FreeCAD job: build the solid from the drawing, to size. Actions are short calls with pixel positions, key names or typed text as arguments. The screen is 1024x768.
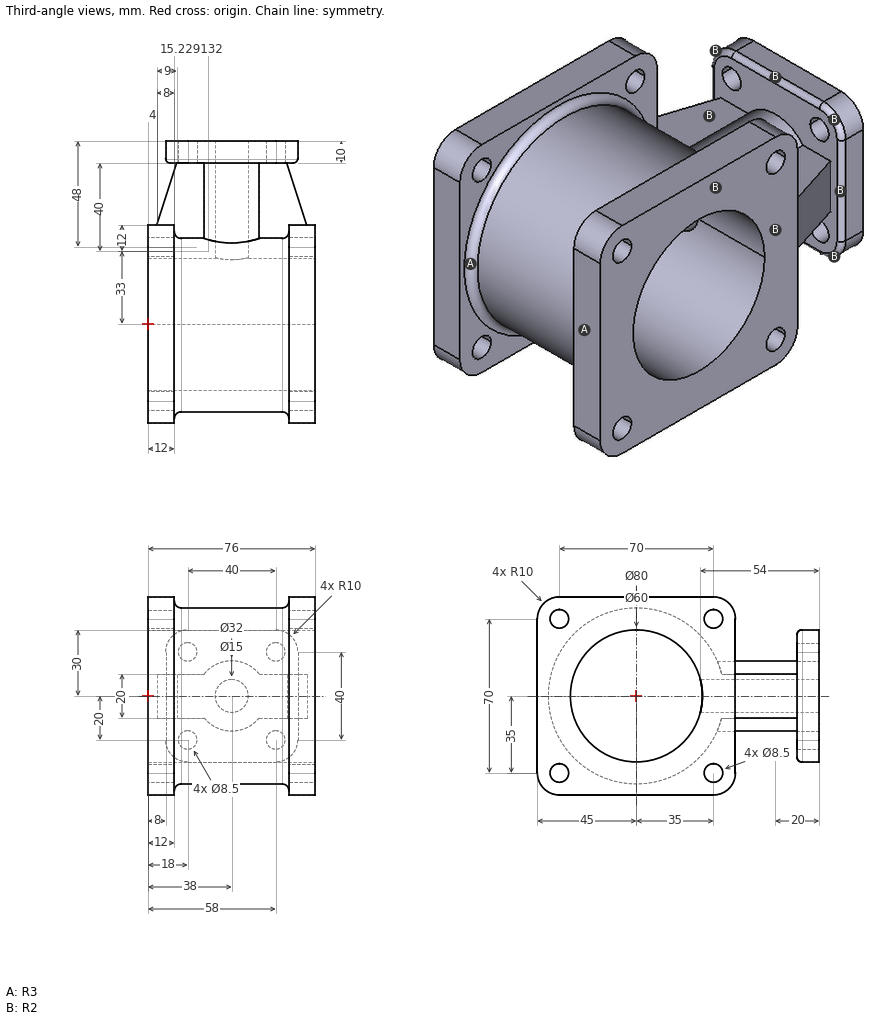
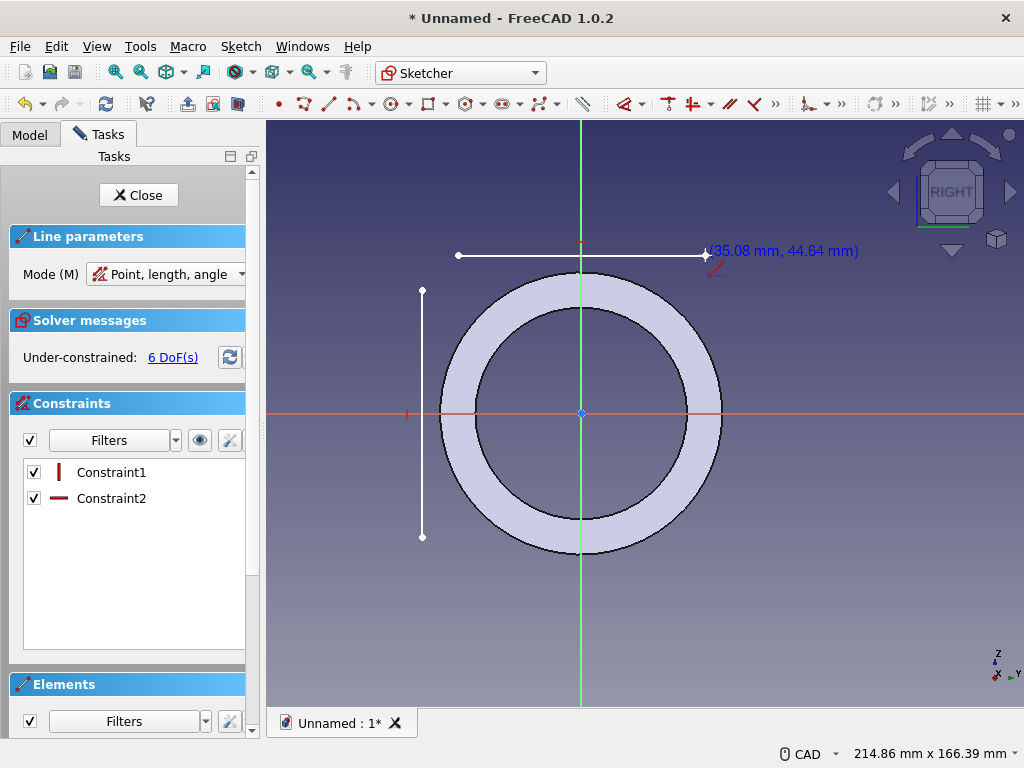
click(740, 290)
click(740, 537)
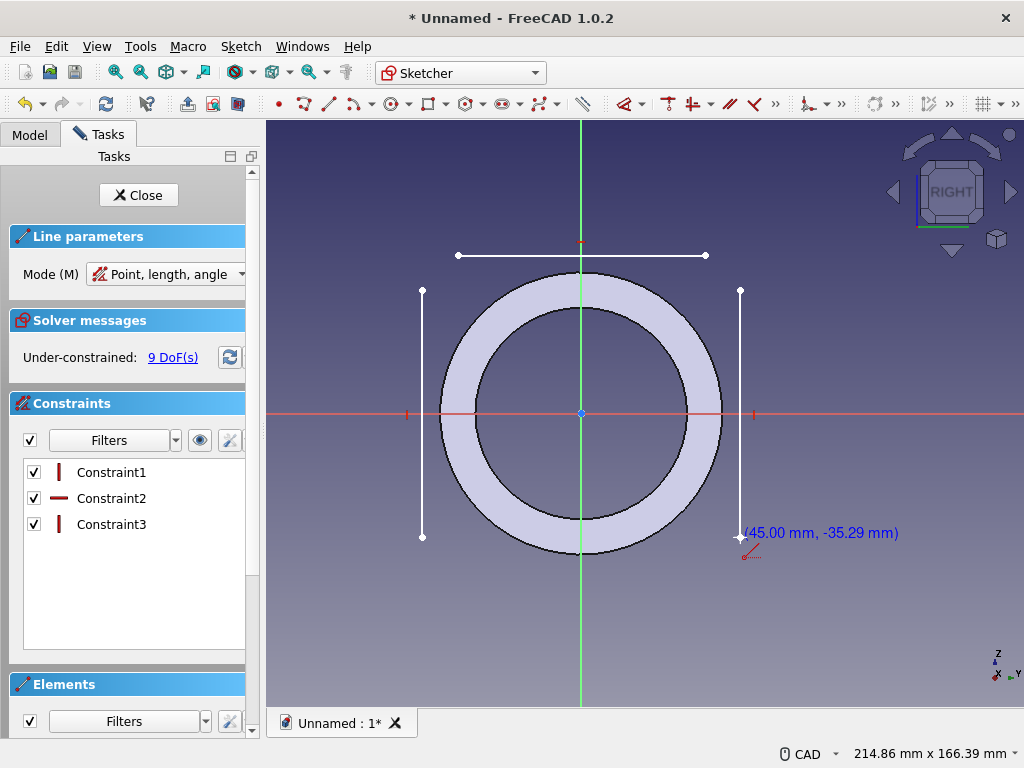
click(705, 572)
click(458, 572)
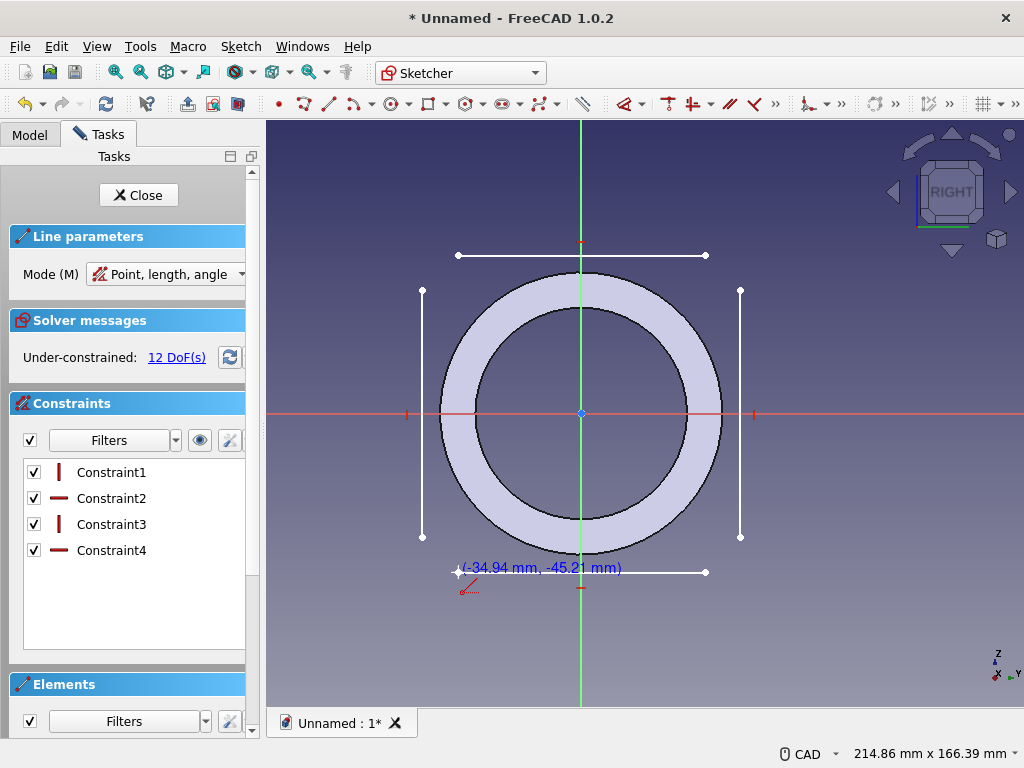
key(g)
key(3)
key(a)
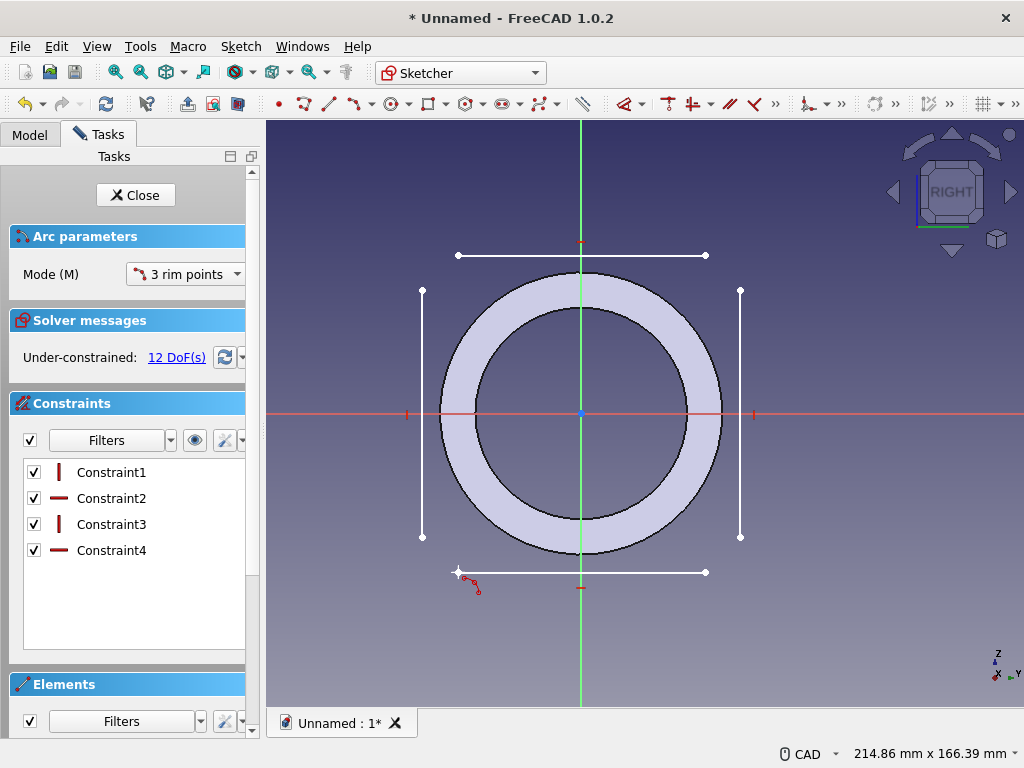
click(422, 291)
click(458, 256)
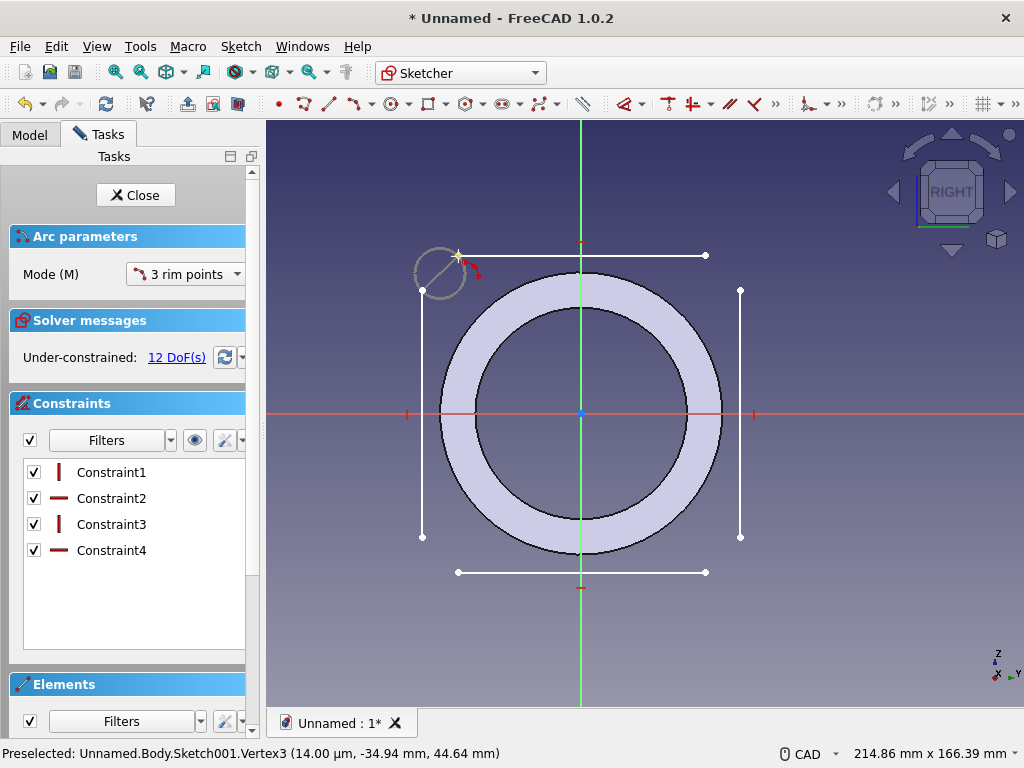
scroll(433, 265, up, 3)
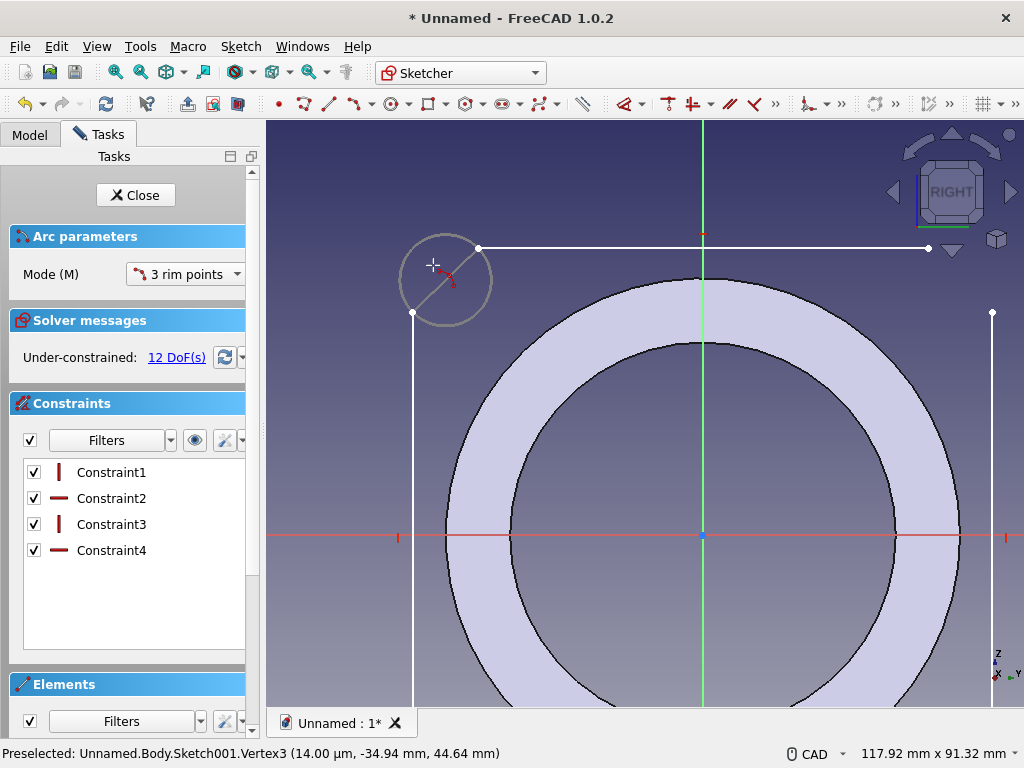
click(432, 265)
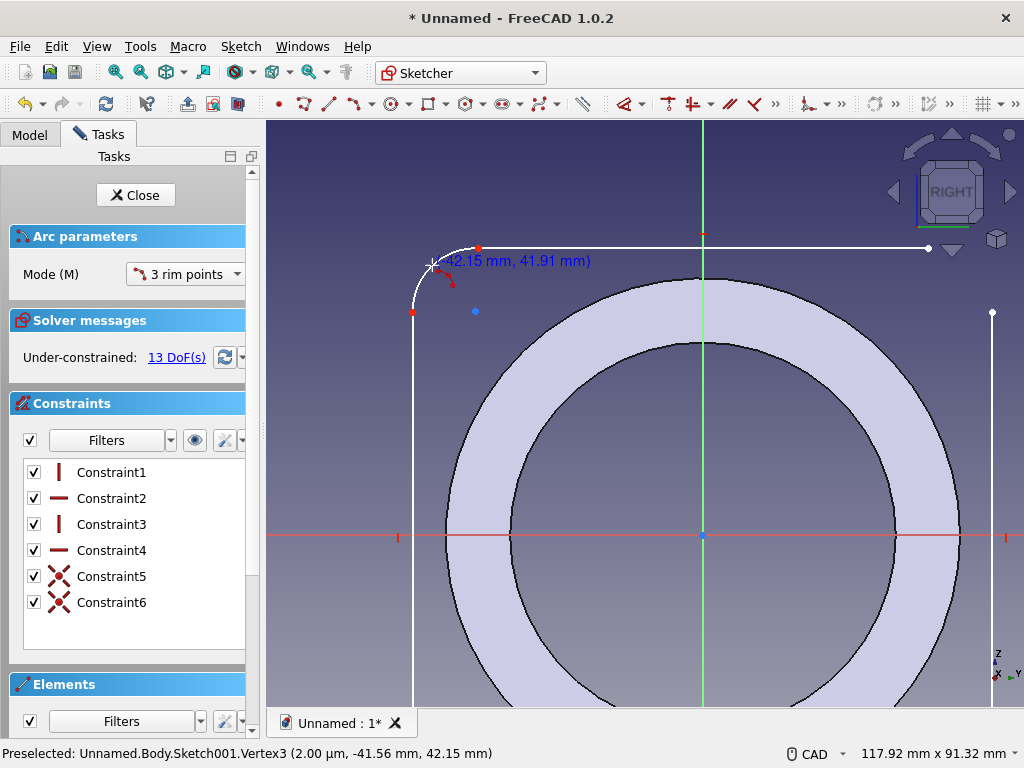
scroll(319, 166, down, 2)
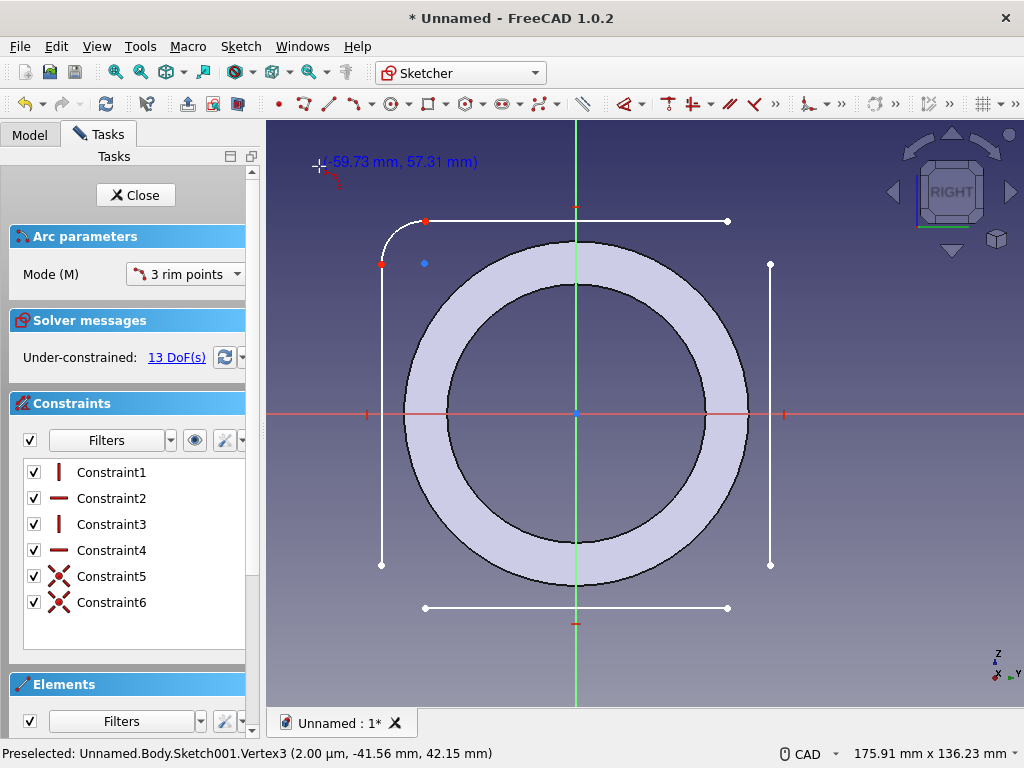
click(728, 221)
click(770, 264)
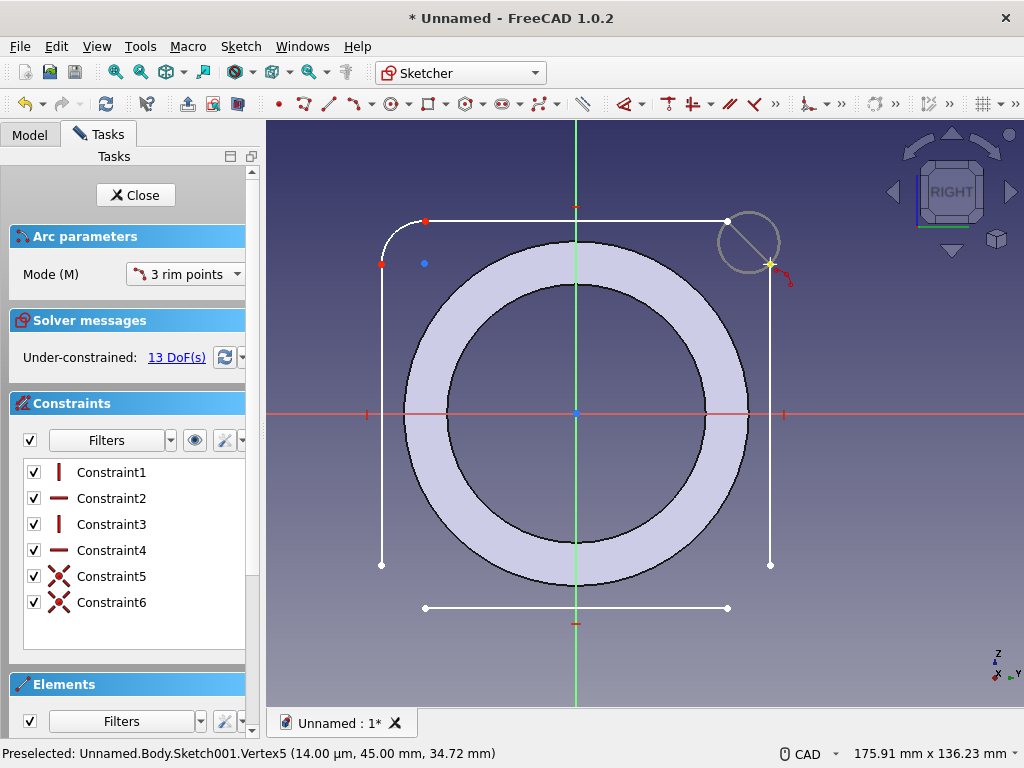
scroll(758, 232, up, 2)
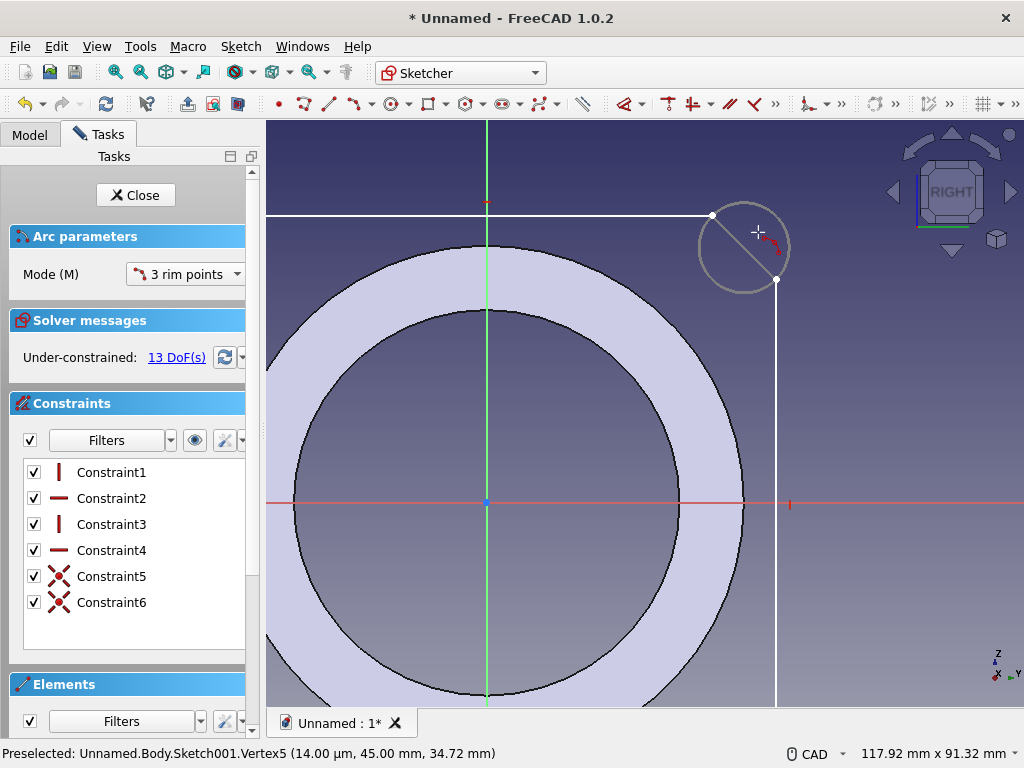
click(757, 232)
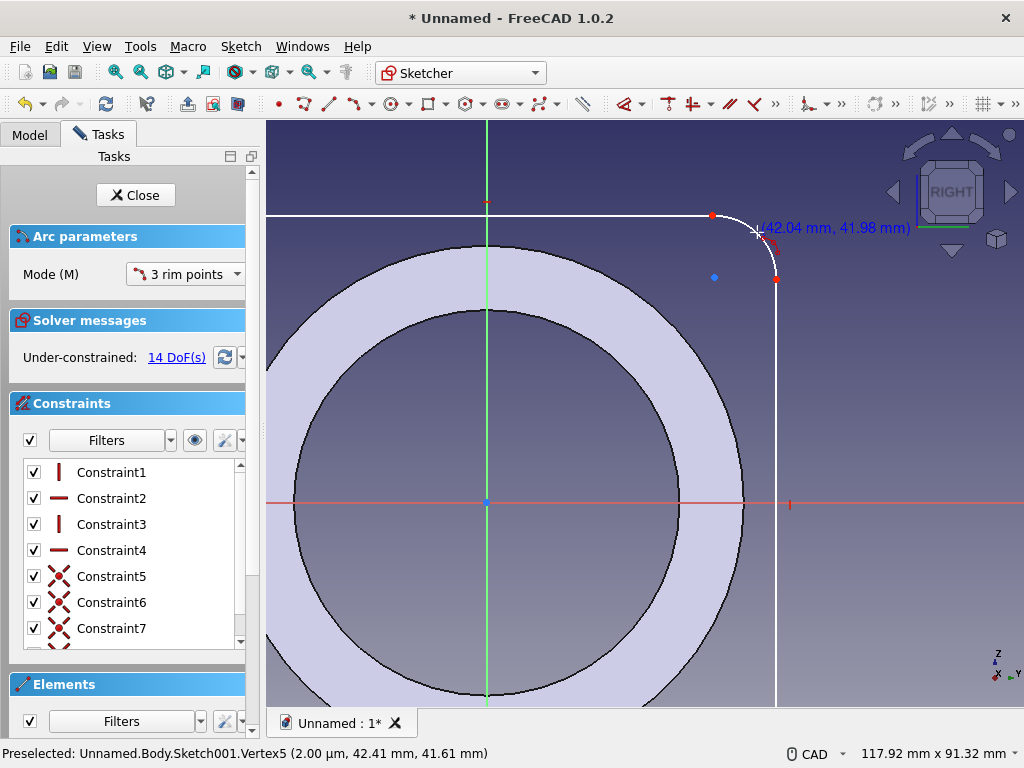
scroll(759, 232, down, 2)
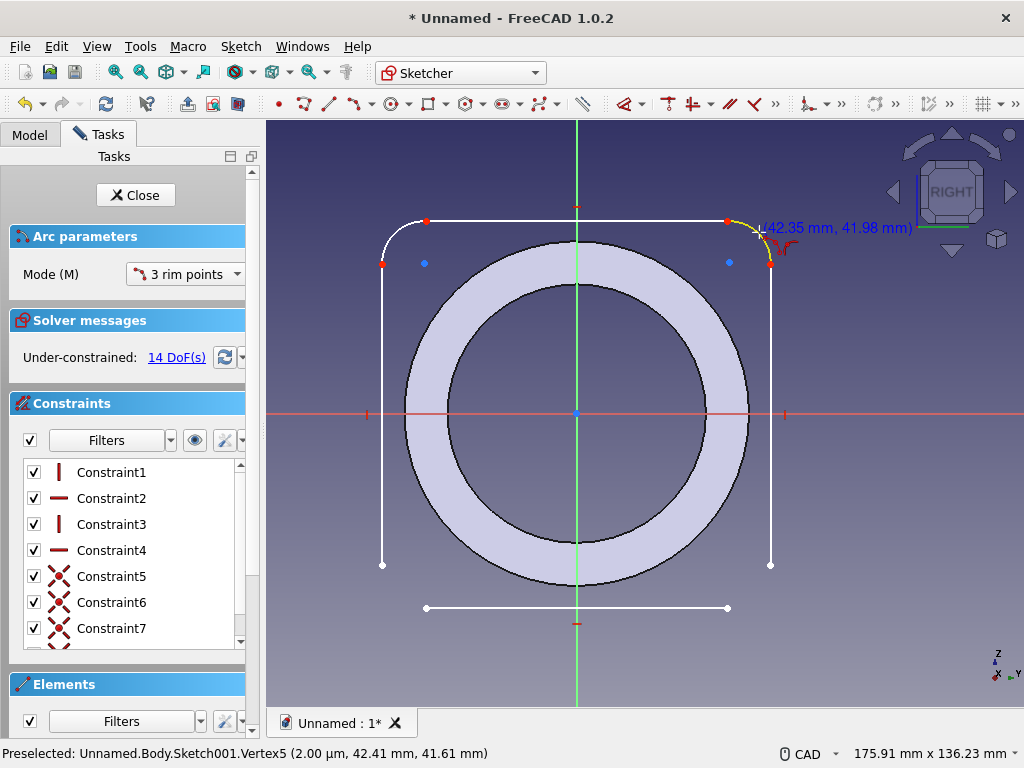
click(771, 566)
click(728, 608)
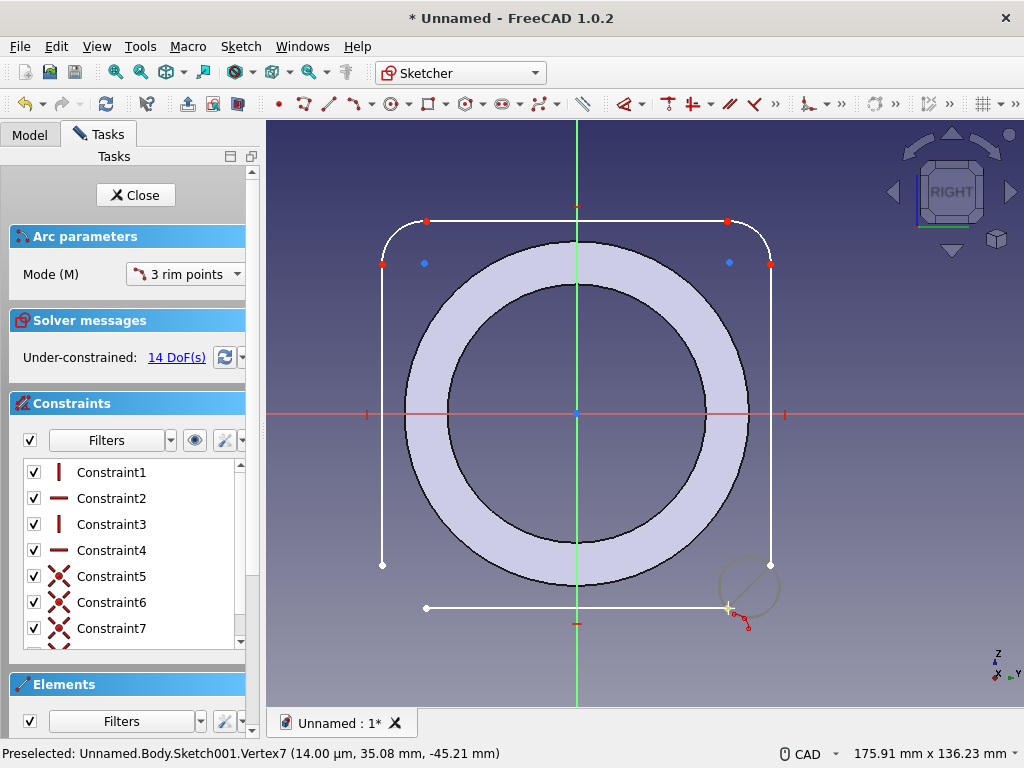
scroll(758, 595, up, 2)